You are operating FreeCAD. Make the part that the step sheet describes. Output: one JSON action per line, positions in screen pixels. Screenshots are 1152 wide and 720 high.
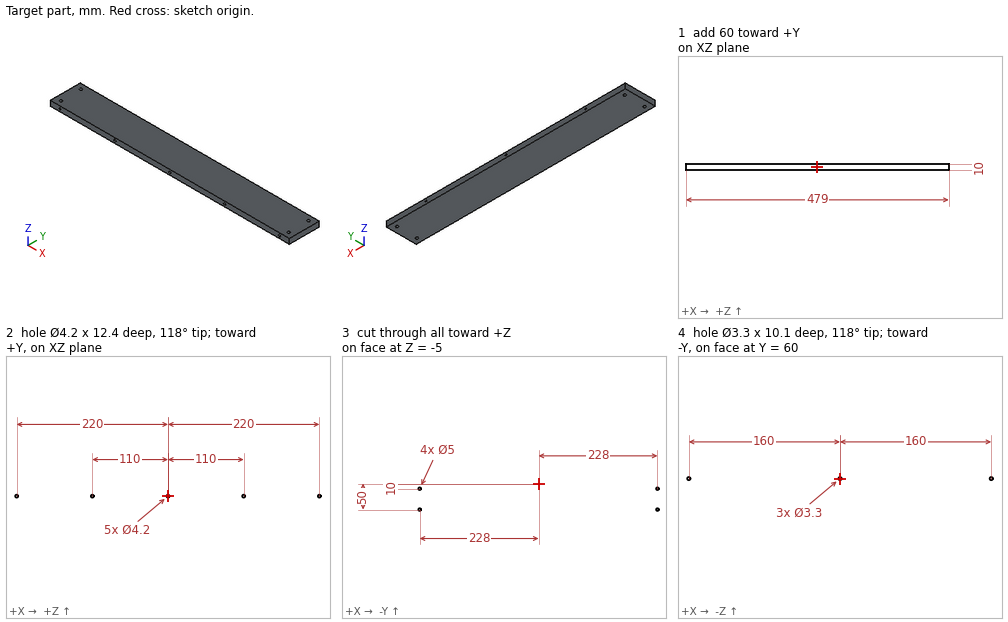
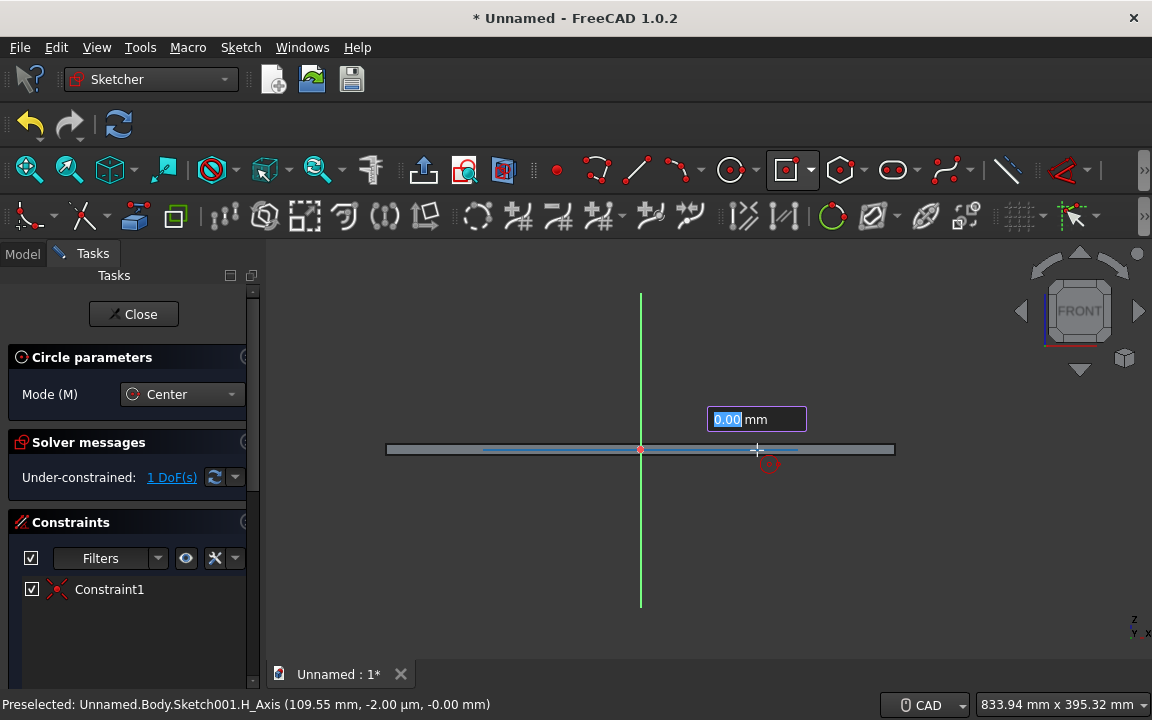
{"action": "scroll", "coordinate": [758, 448], "scroll_direction": "up", "scroll_amount": 11}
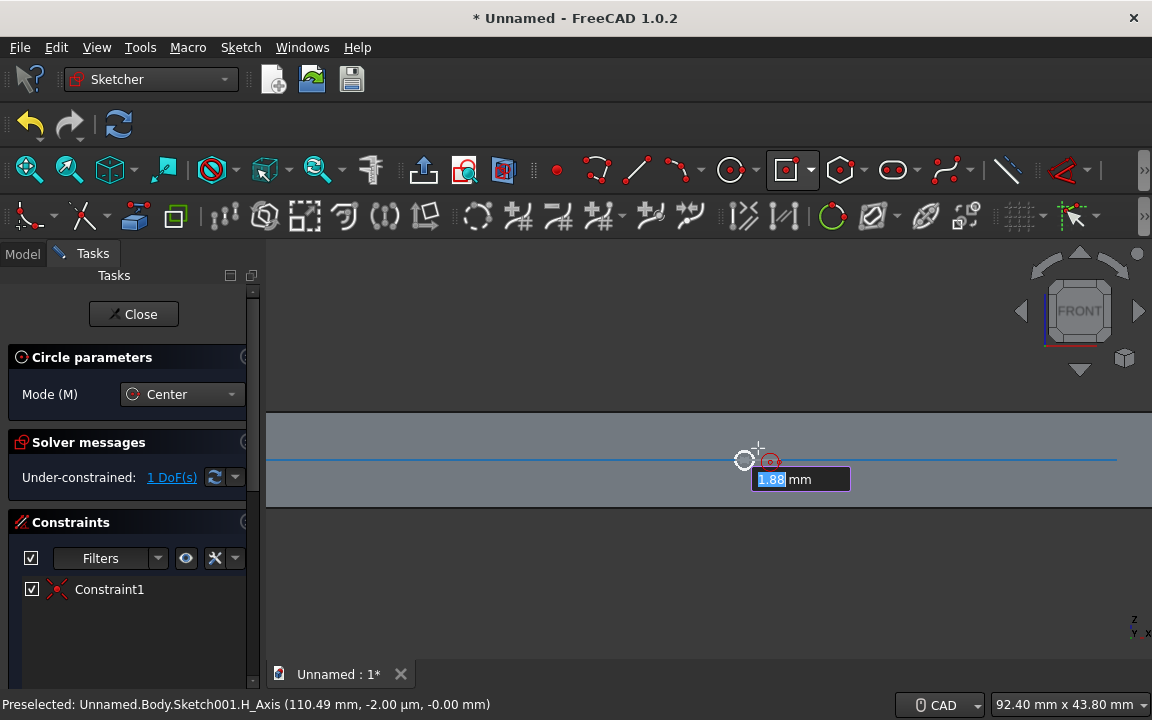
{"action": "left_click", "coordinate": [756, 441]}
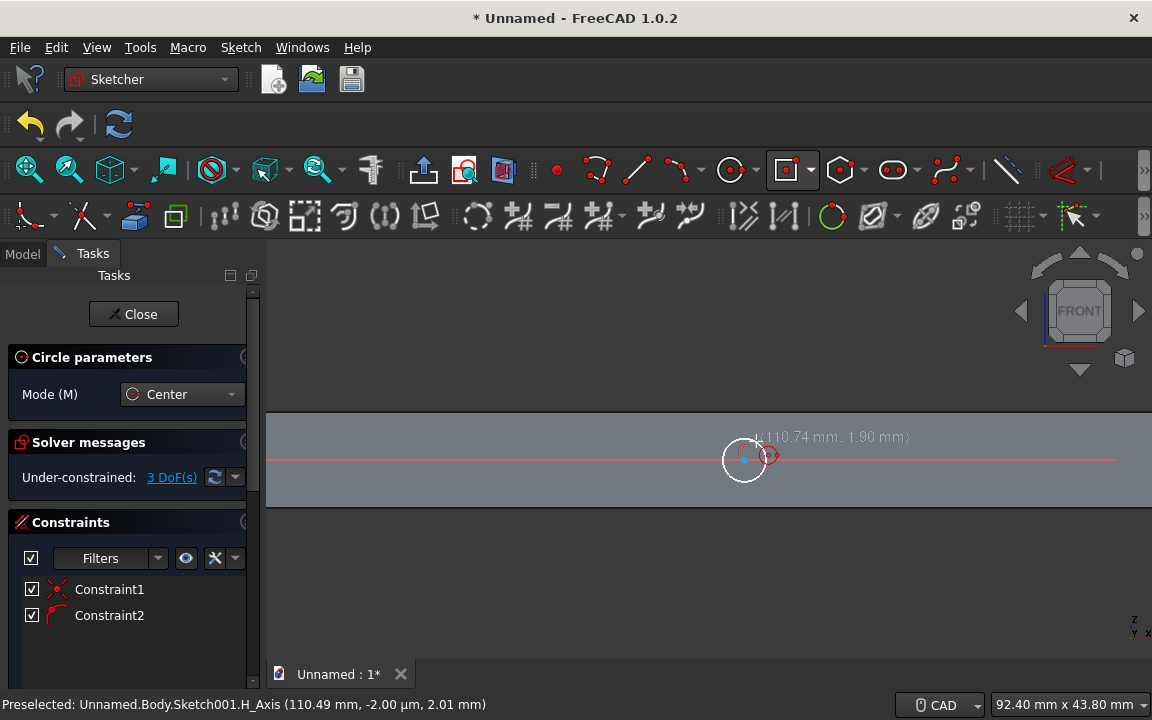
{"action": "scroll", "coordinate": [758, 448], "scroll_direction": "down", "scroll_amount": 11}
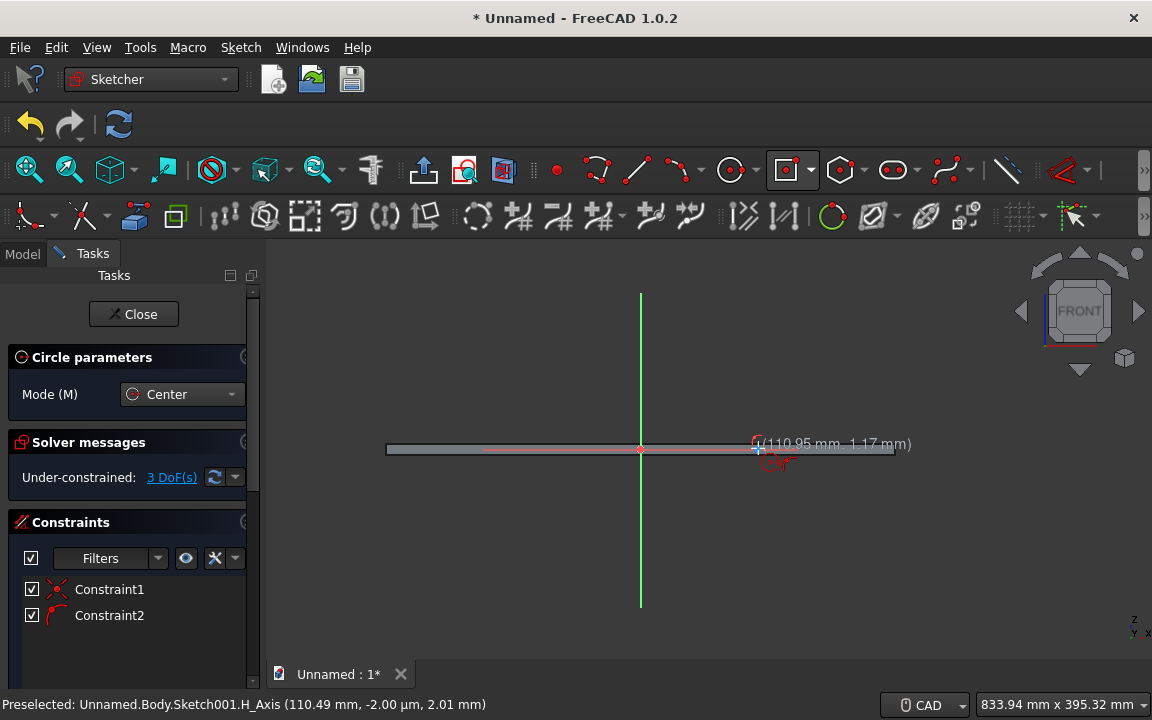
{"action": "scroll", "coordinate": [874, 450], "scroll_direction": "up", "scroll_amount": 12}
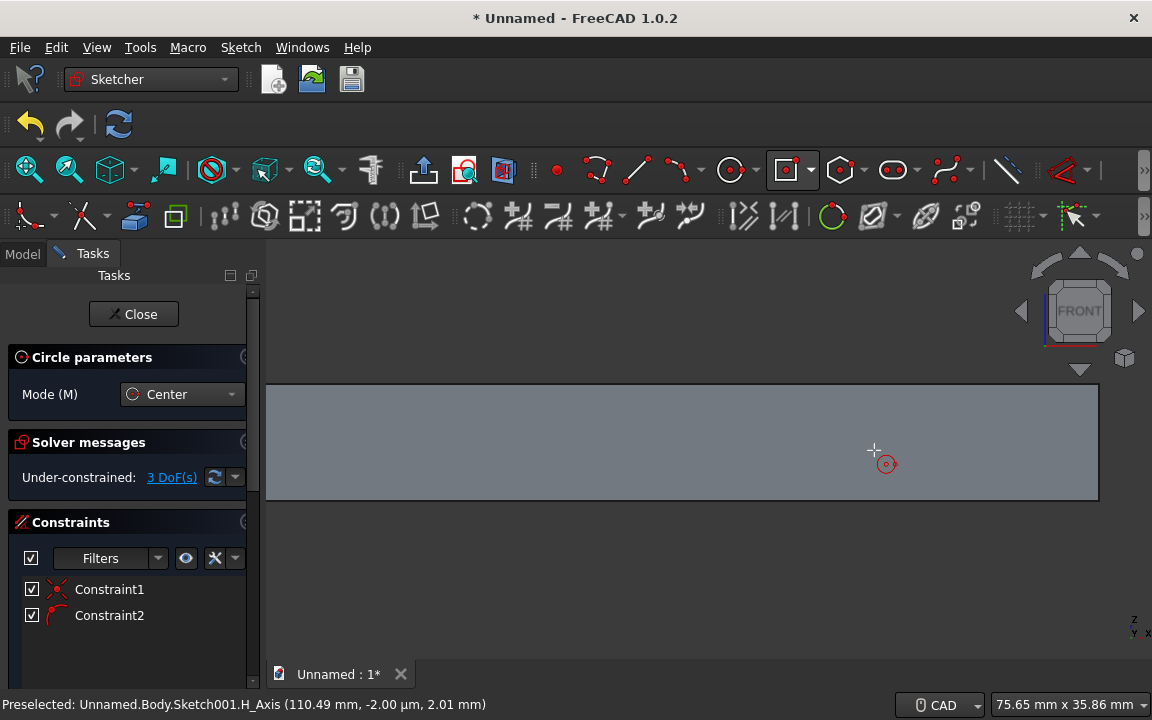
{"action": "scroll", "coordinate": [875, 450], "scroll_direction": "down", "scroll_amount": 12}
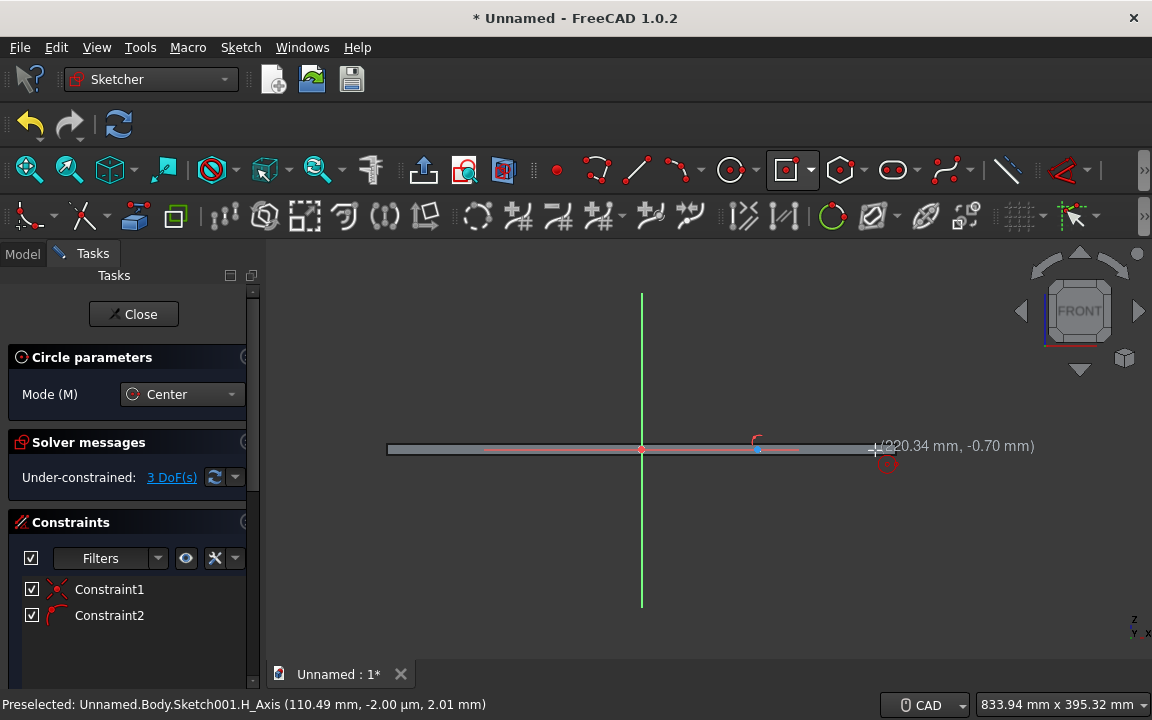
{"action": "left_click", "coordinate": [875, 450]}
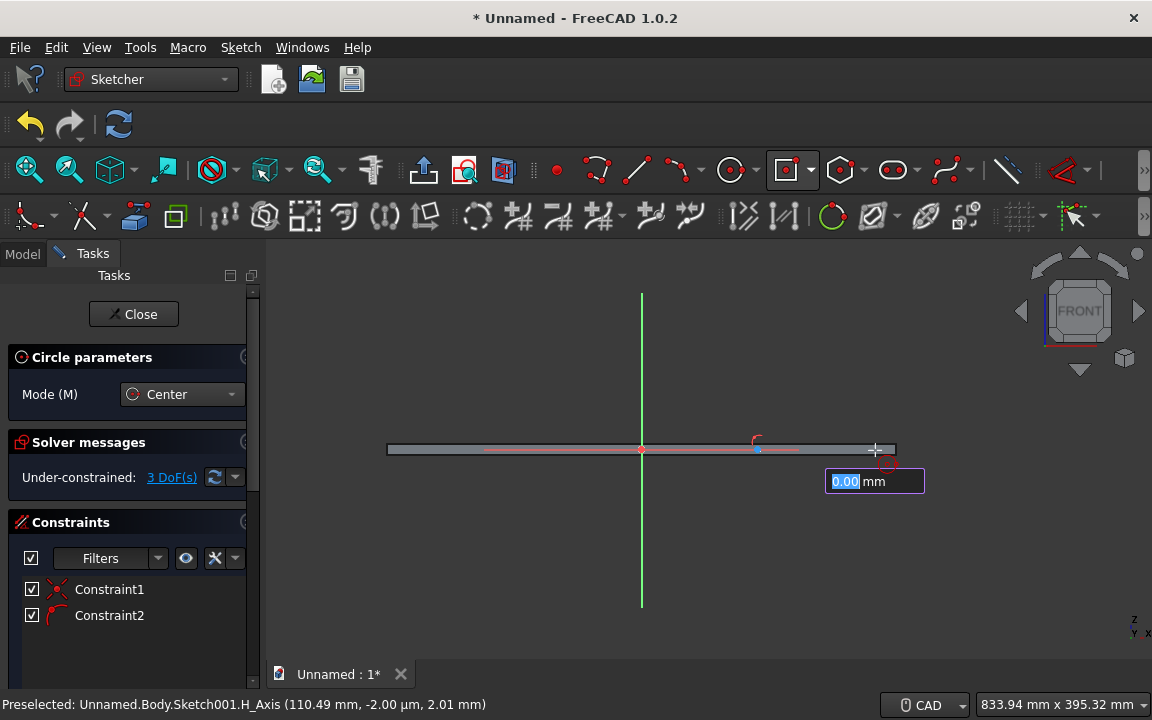
{"action": "scroll", "coordinate": [874, 452], "scroll_direction": "up", "scroll_amount": 11}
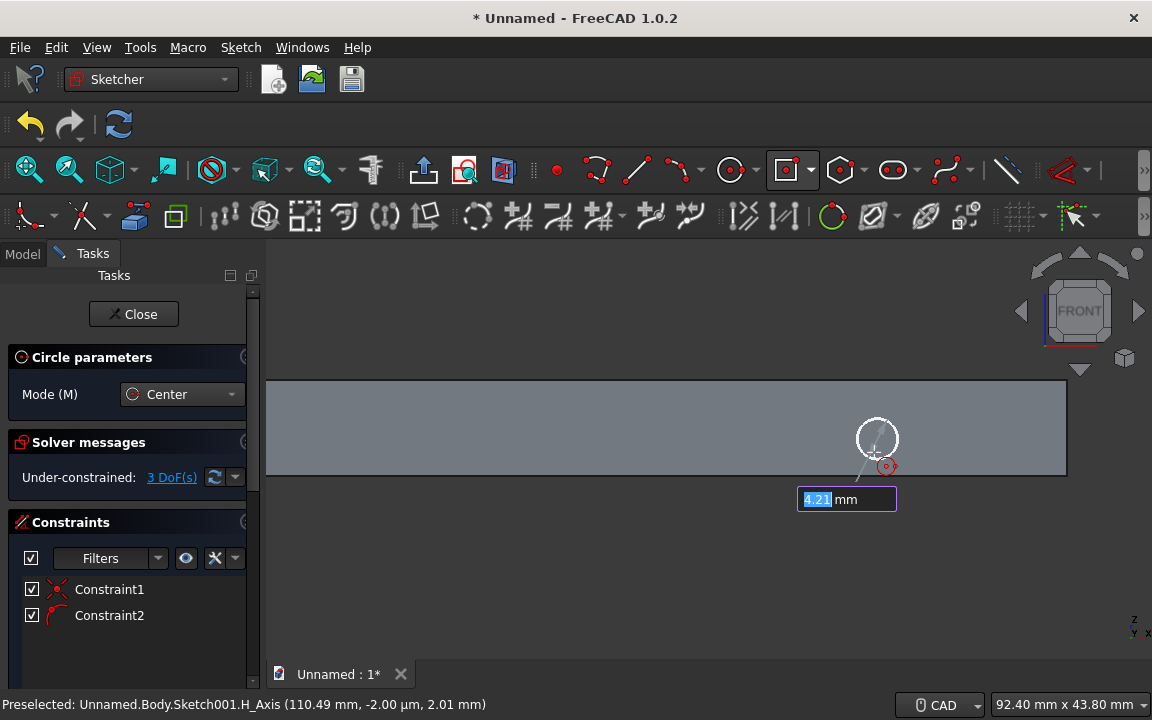
{"action": "left_click", "coordinate": [873, 447]}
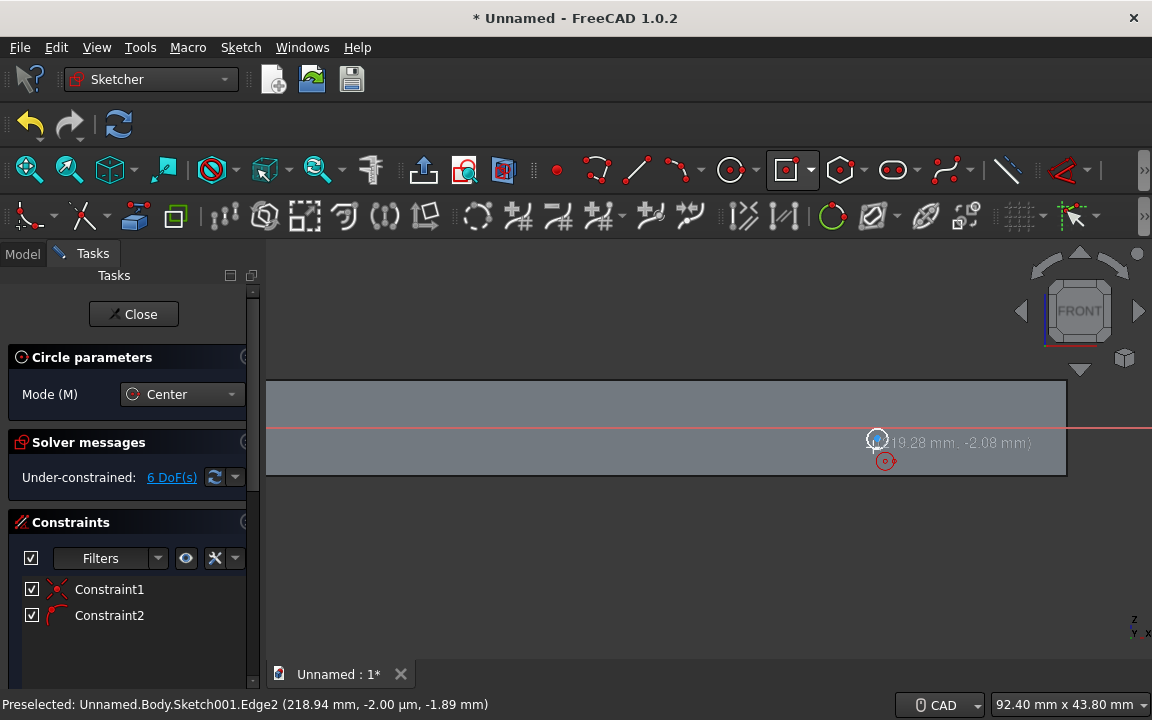
{"action": "scroll", "coordinate": [874, 452], "scroll_direction": "down", "scroll_amount": 11}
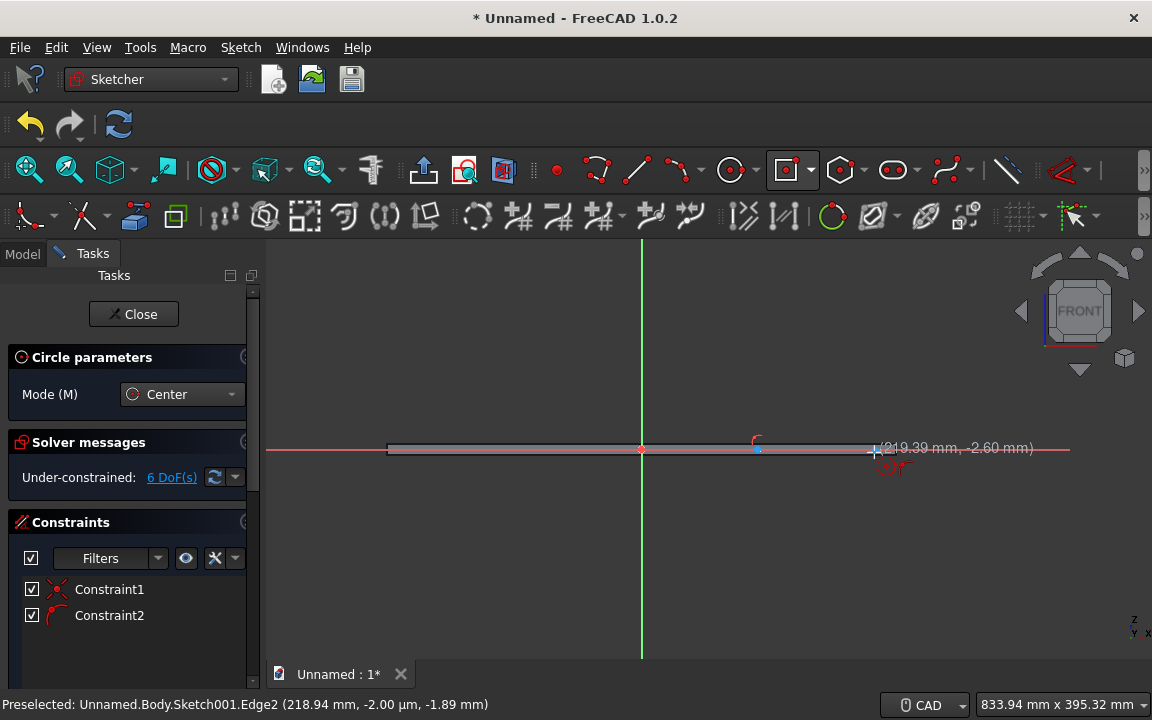
{"action": "scroll", "coordinate": [408, 450], "scroll_direction": "up", "scroll_amount": 12}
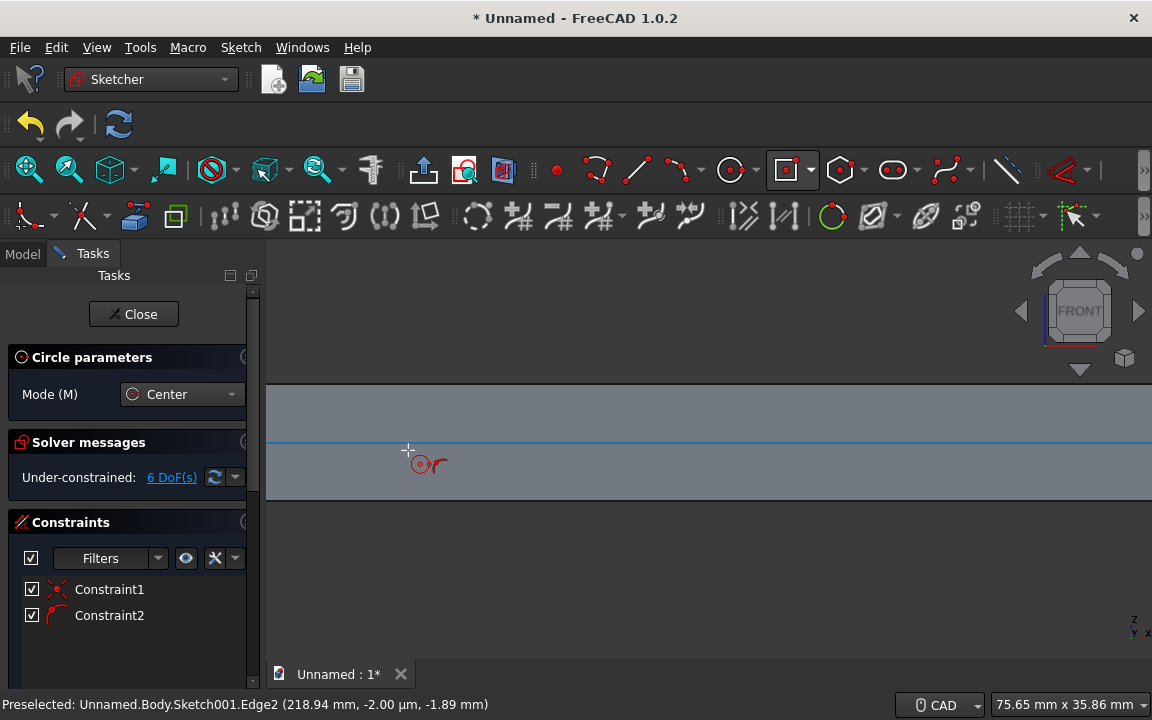
{"action": "scroll", "coordinate": [407, 450], "scroll_direction": "down", "scroll_amount": 12}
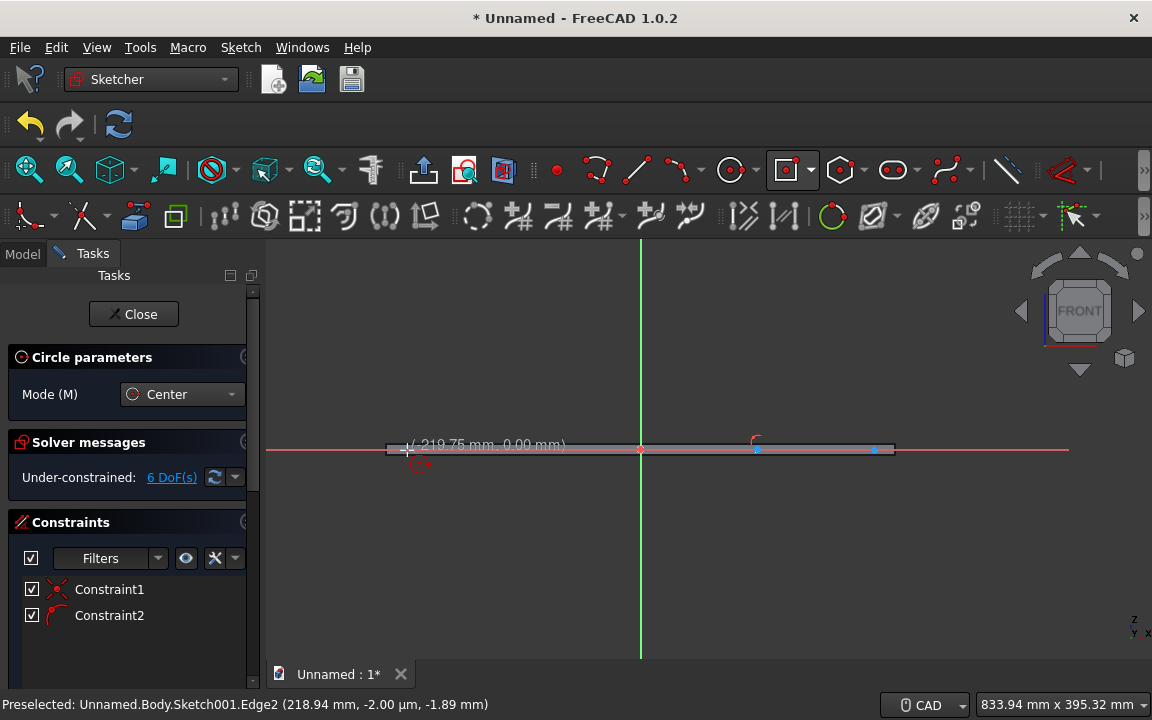
{"action": "left_click", "coordinate": [407, 450]}